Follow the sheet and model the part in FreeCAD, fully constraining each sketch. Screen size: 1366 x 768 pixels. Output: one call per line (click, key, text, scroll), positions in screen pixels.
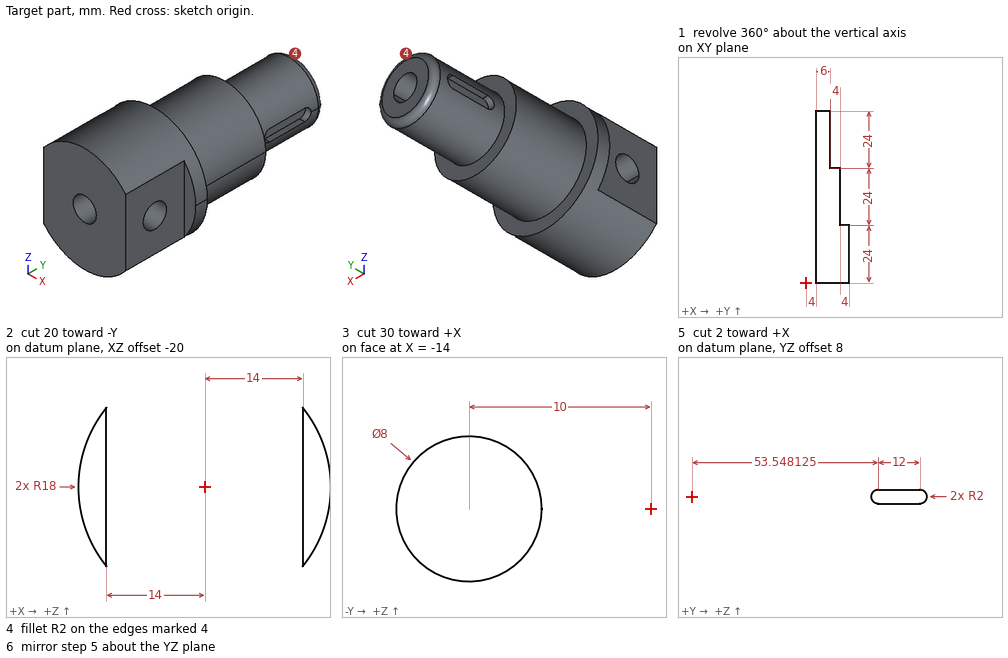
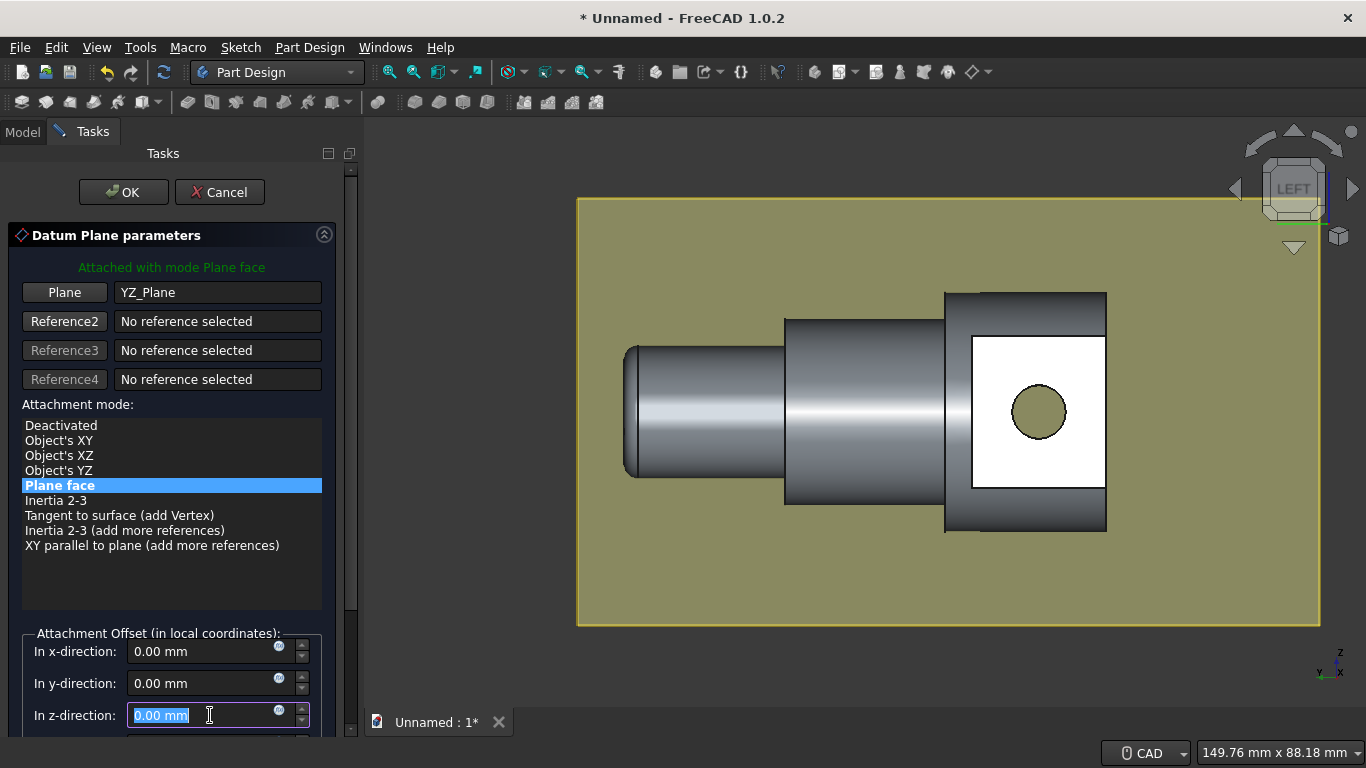
text(8)
key(Tab)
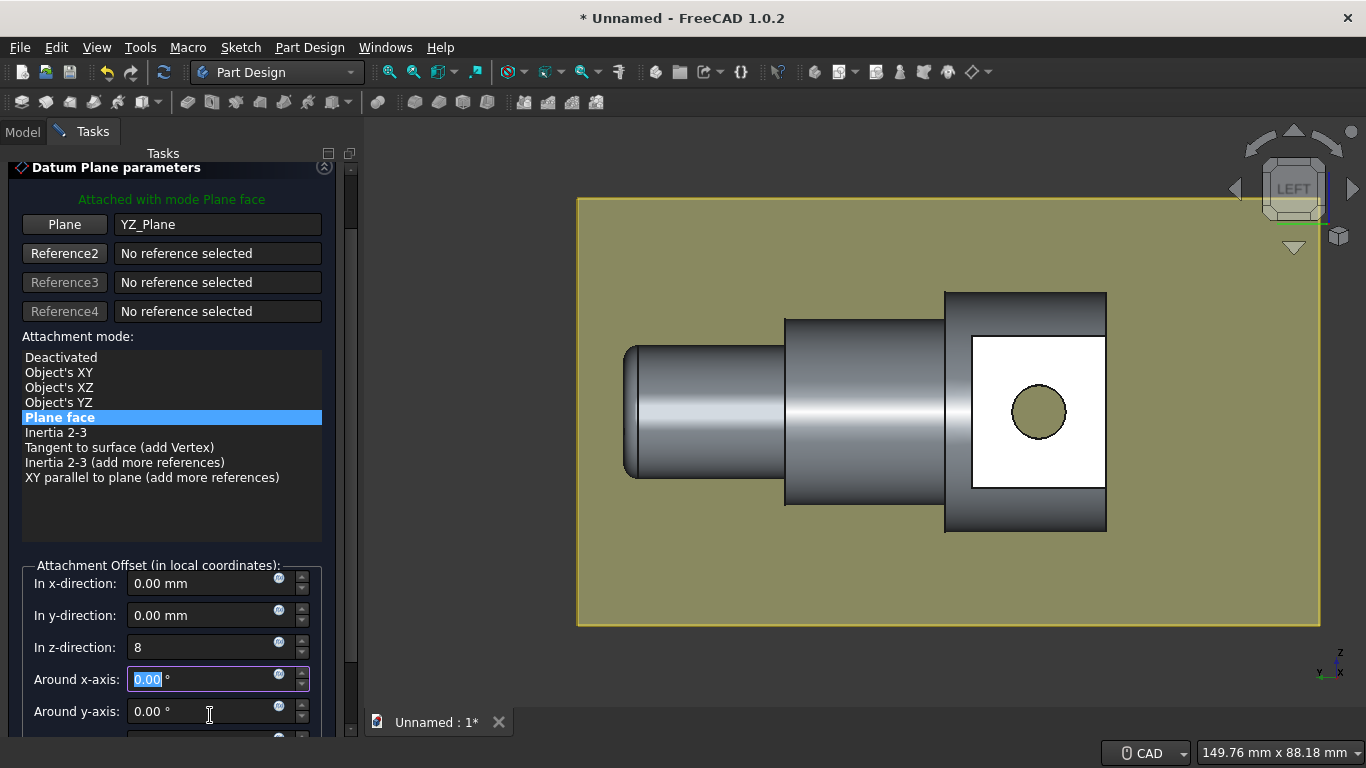
scroll(351, 450, up, 2)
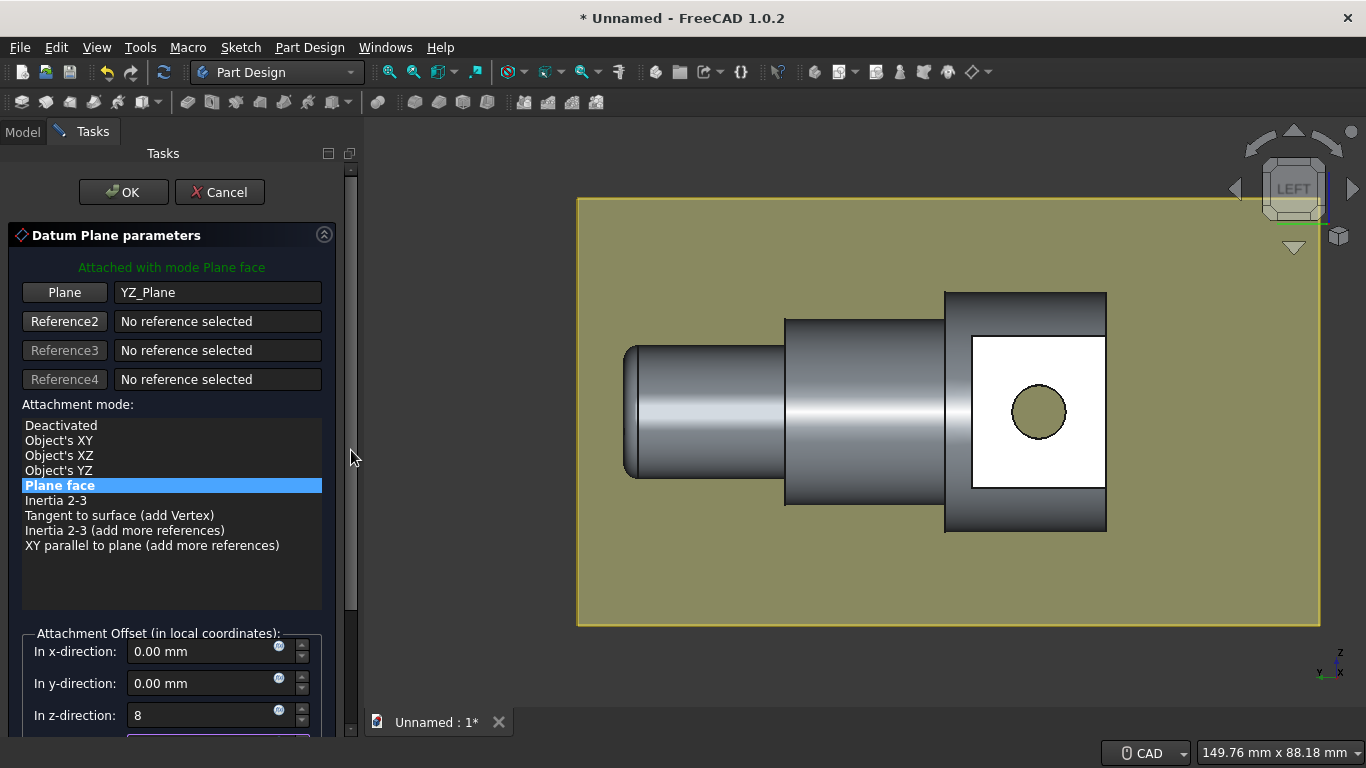
click(124, 192)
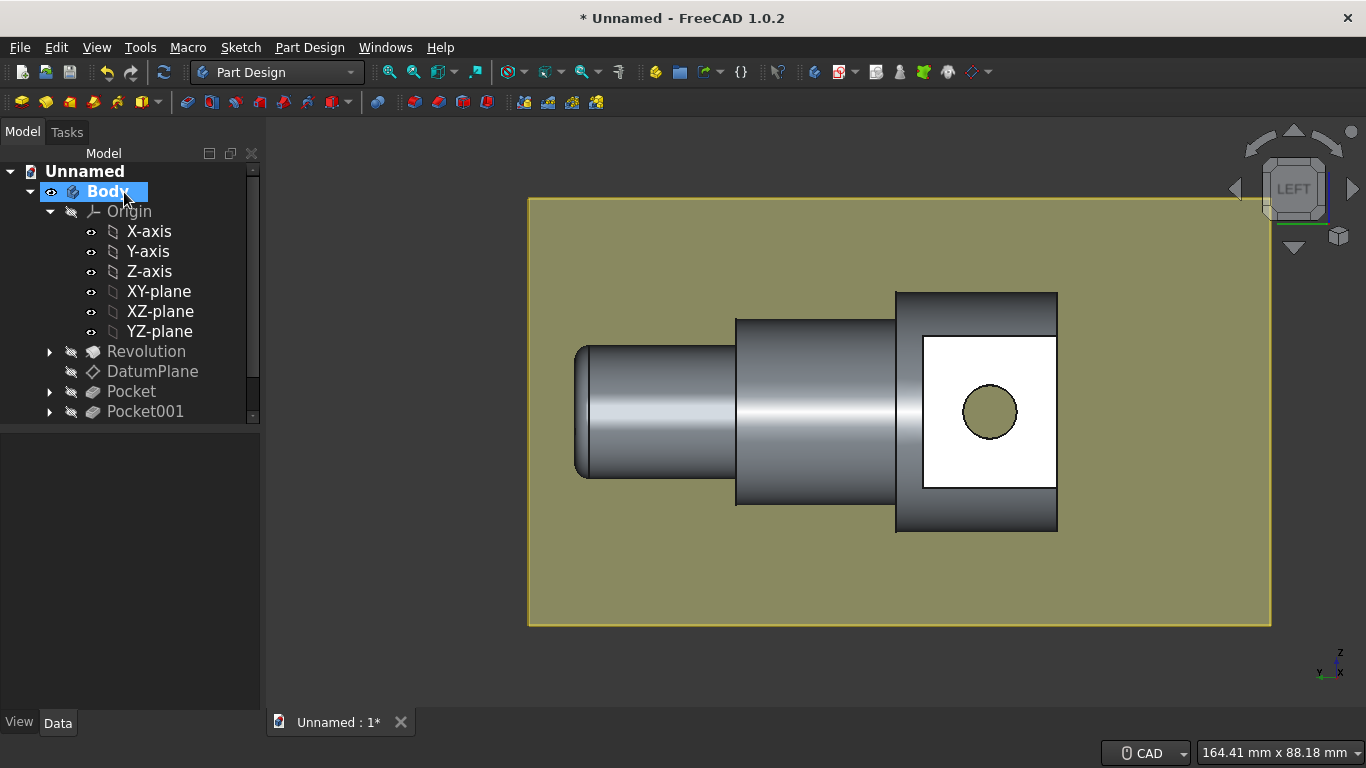
scroll(100, 287, down, 3)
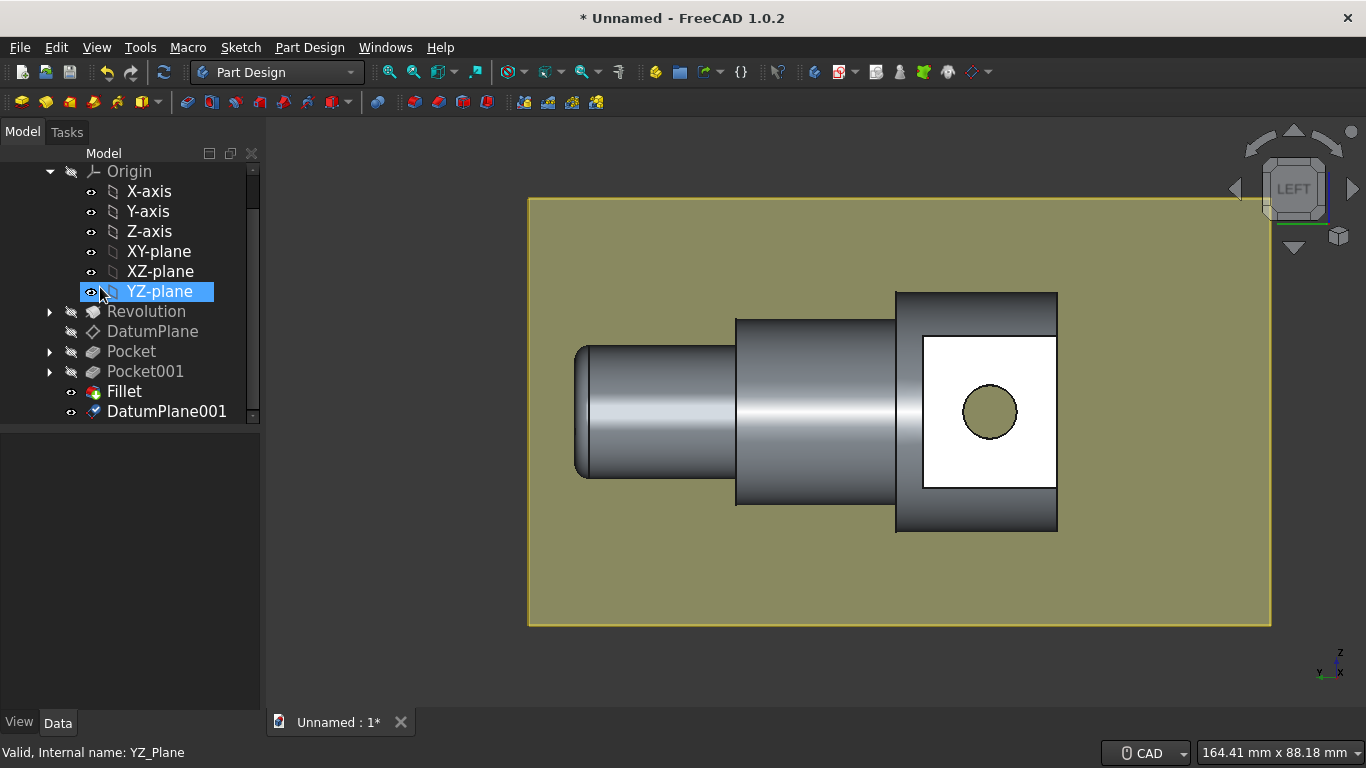
click(116, 412)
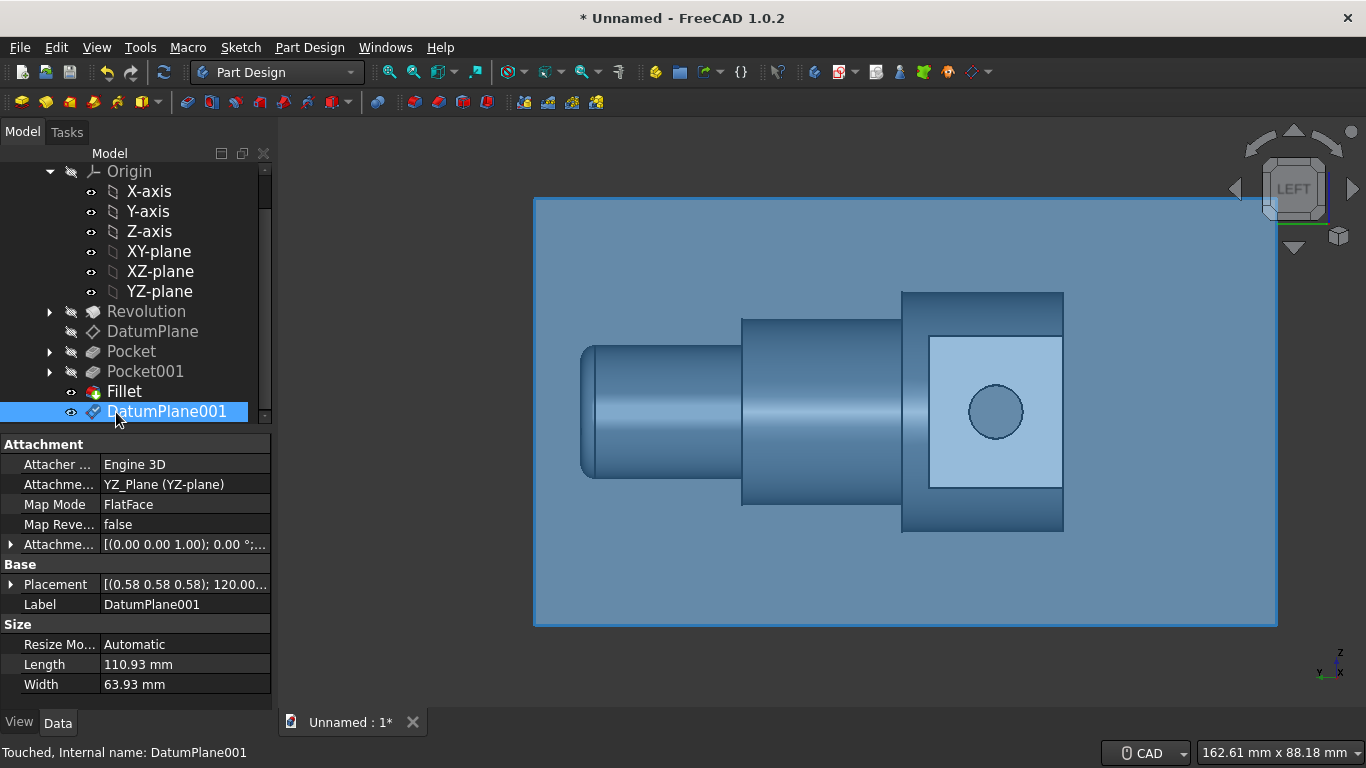
click(840, 72)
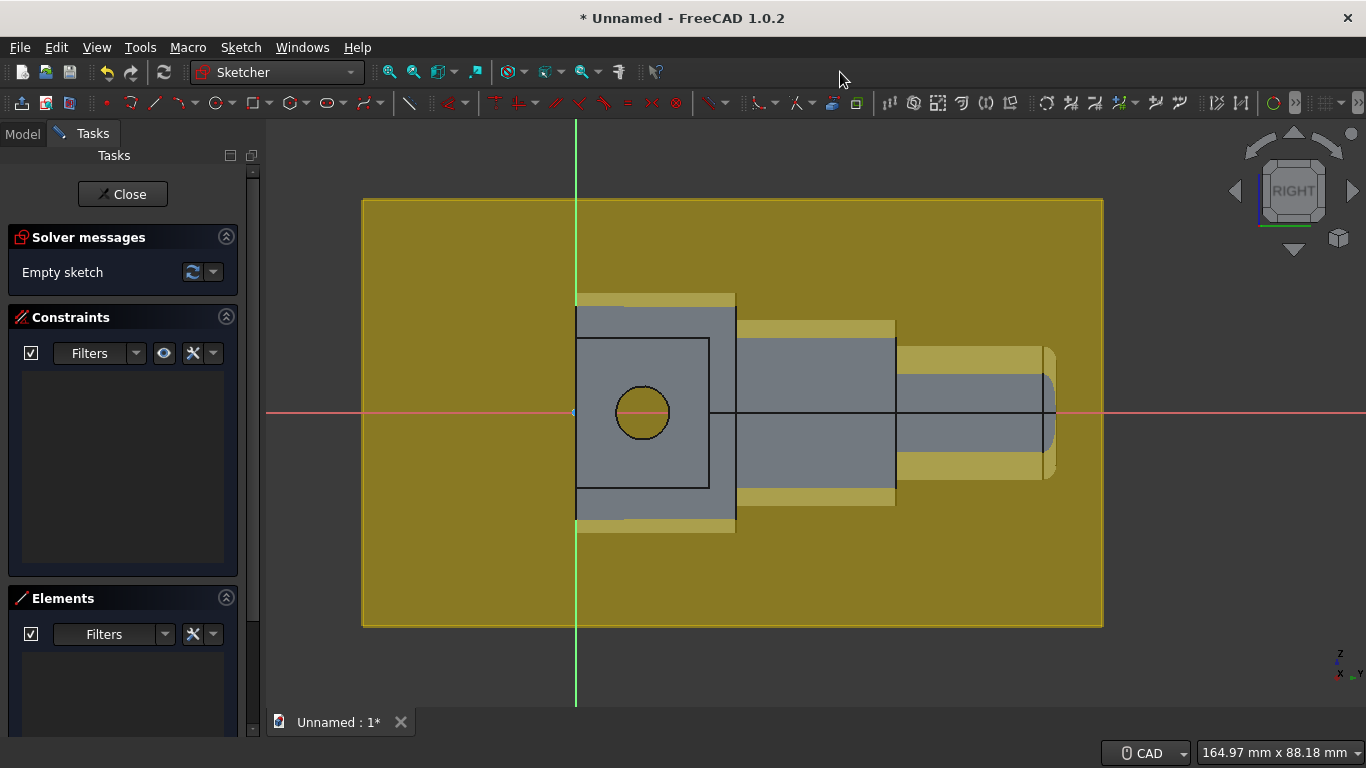
click(70, 104)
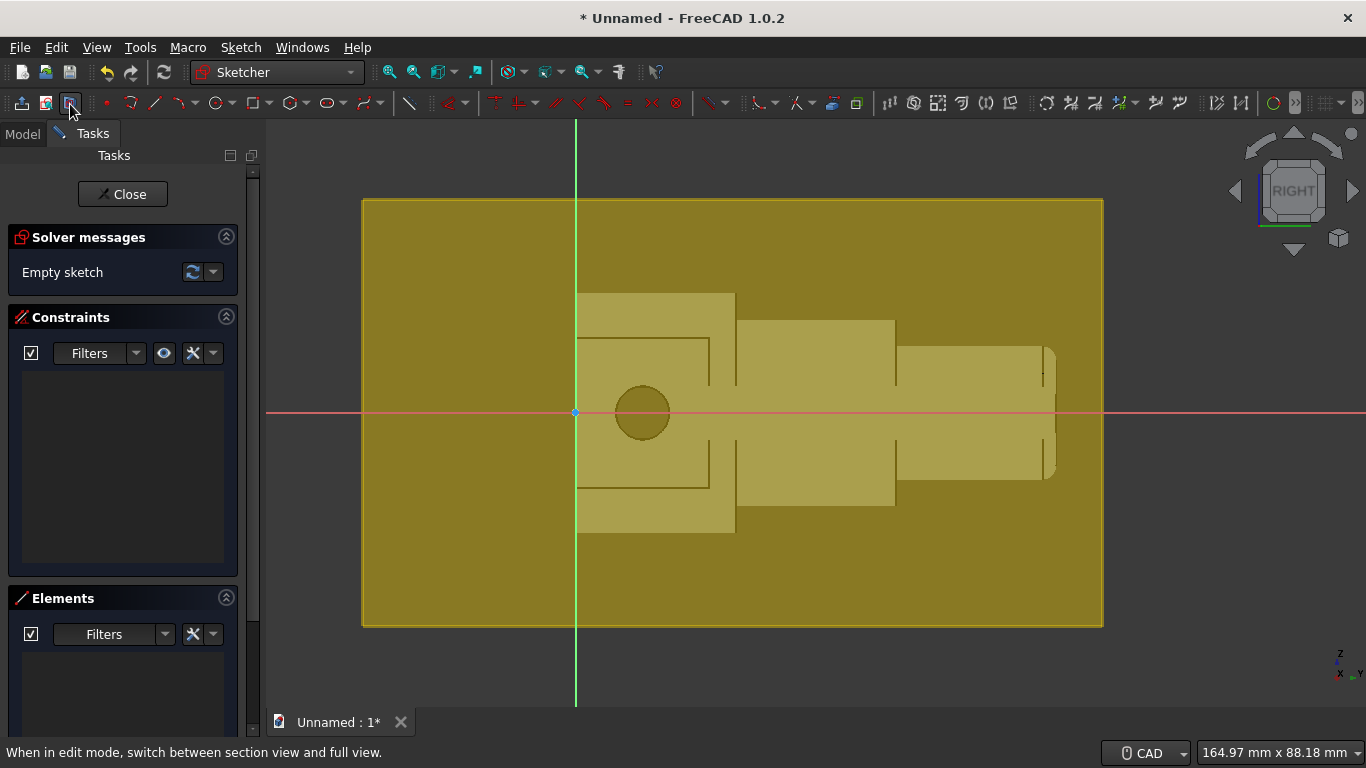
scroll(1018, 413, up, 9)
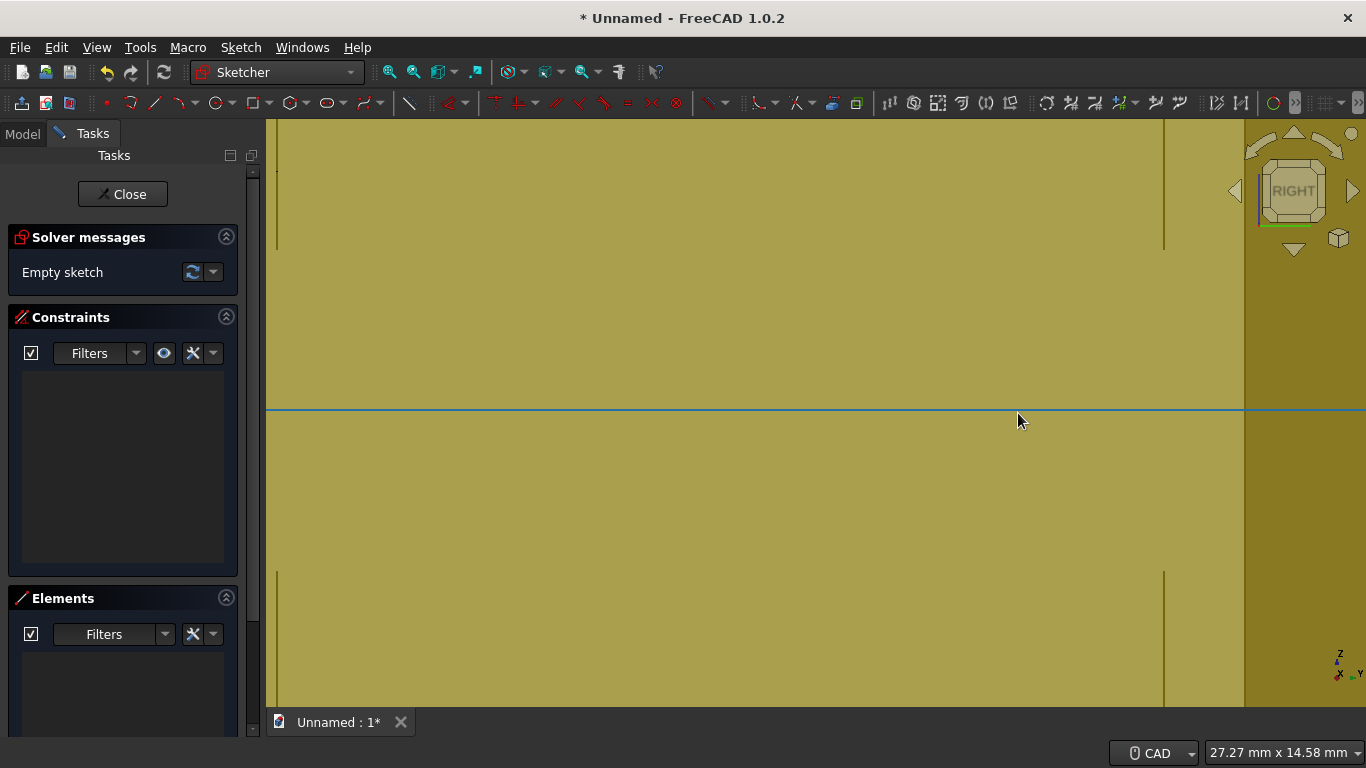
click(328, 104)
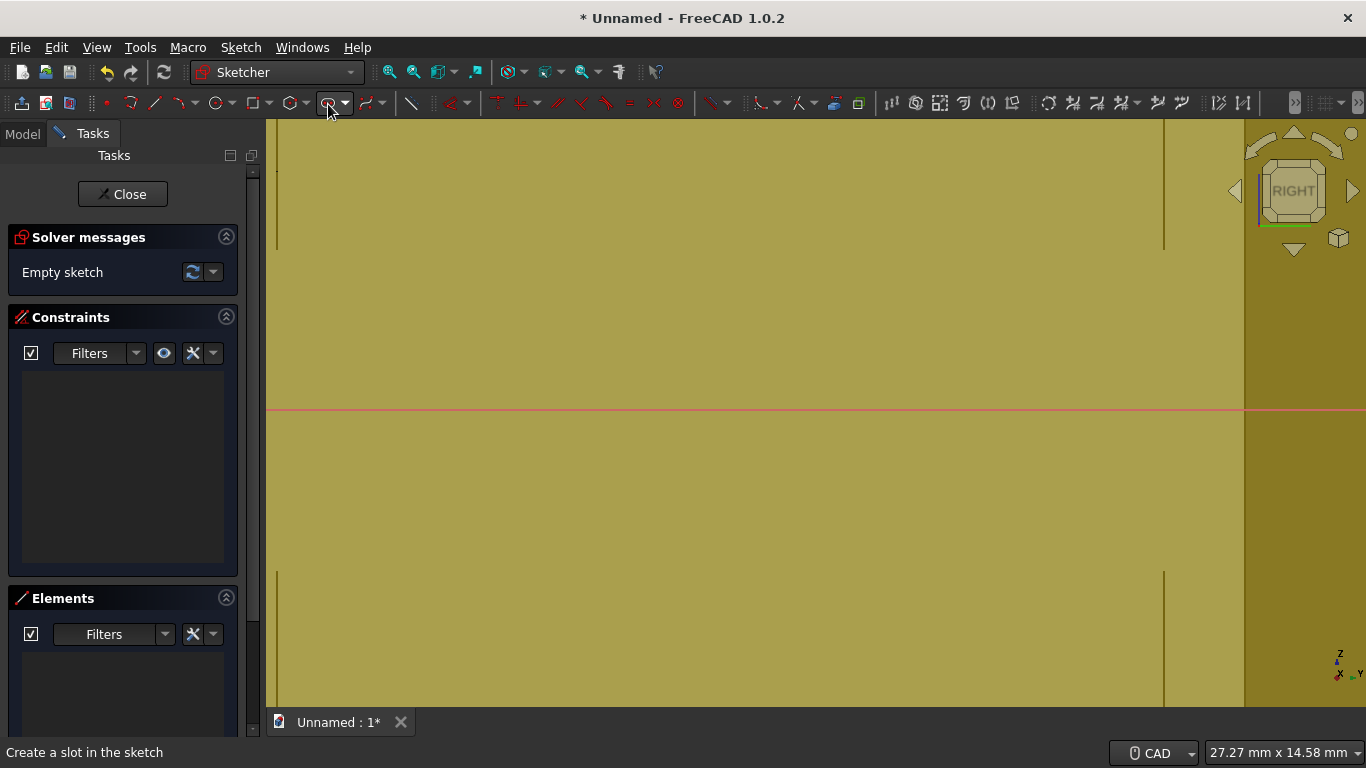
click(500, 410)